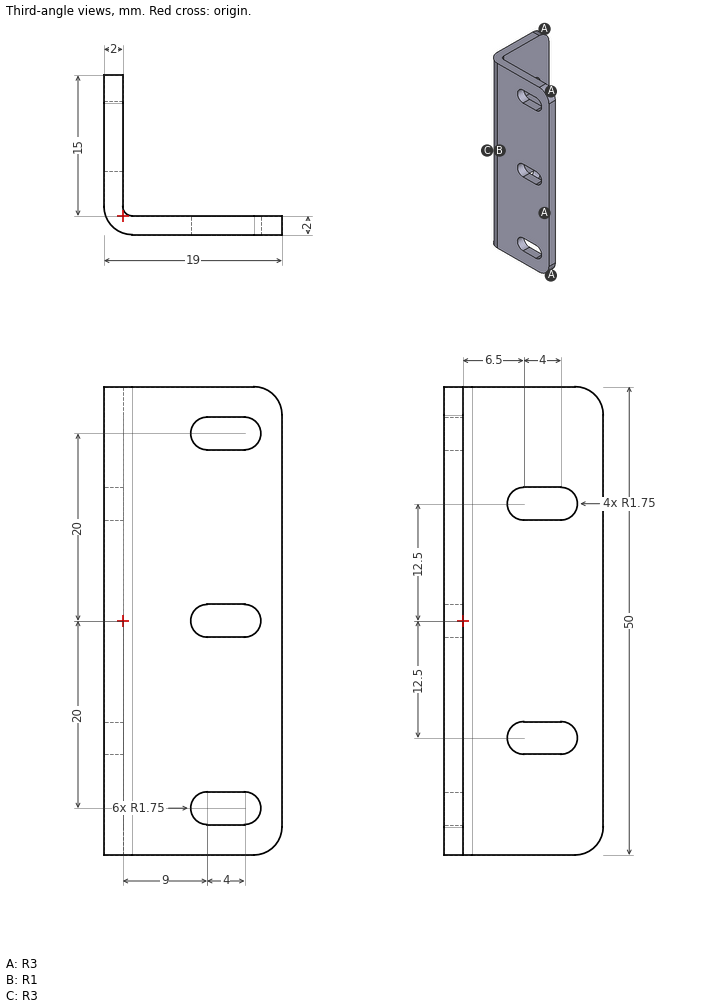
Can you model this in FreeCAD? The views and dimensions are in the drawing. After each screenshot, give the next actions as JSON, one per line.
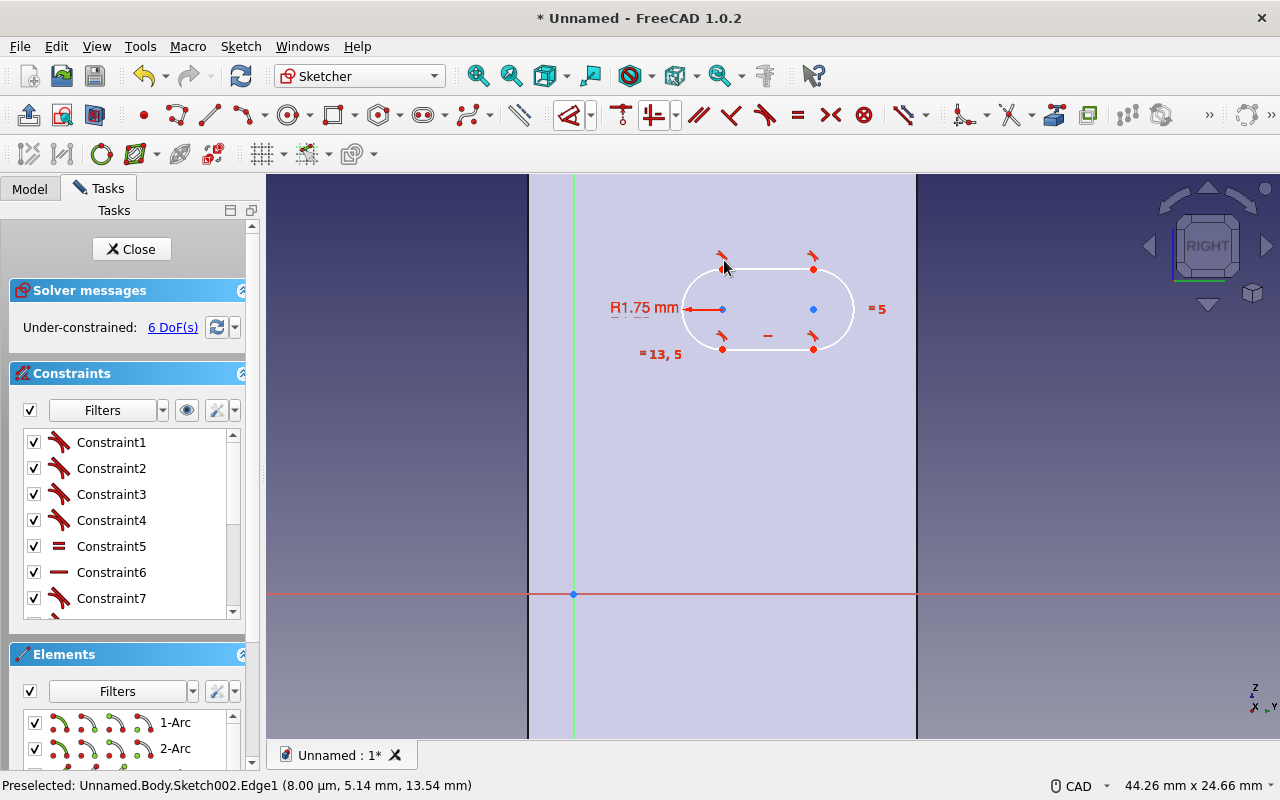
{"action": "left_click", "coordinate": [750, 269]}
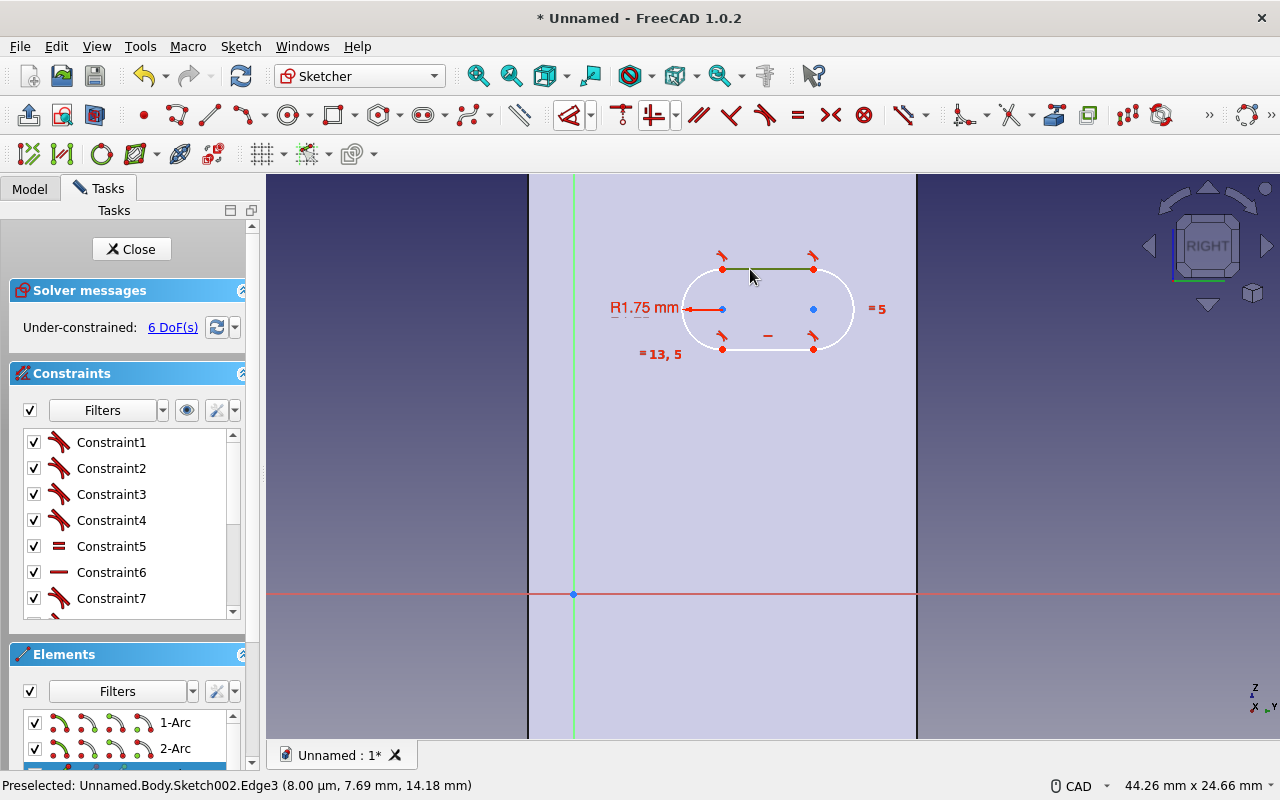
{"action": "left_click", "coordinate": [590, 116]}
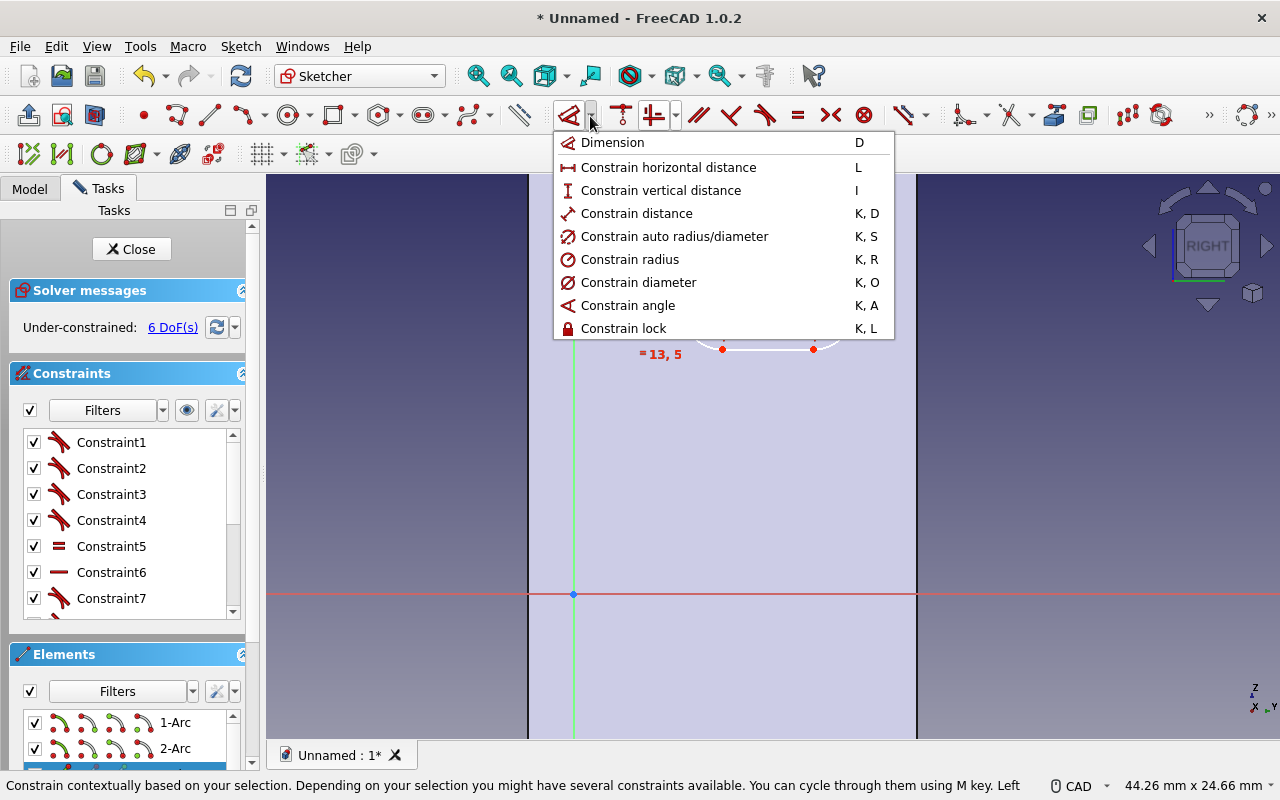
{"action": "left_click", "coordinate": [724, 168]}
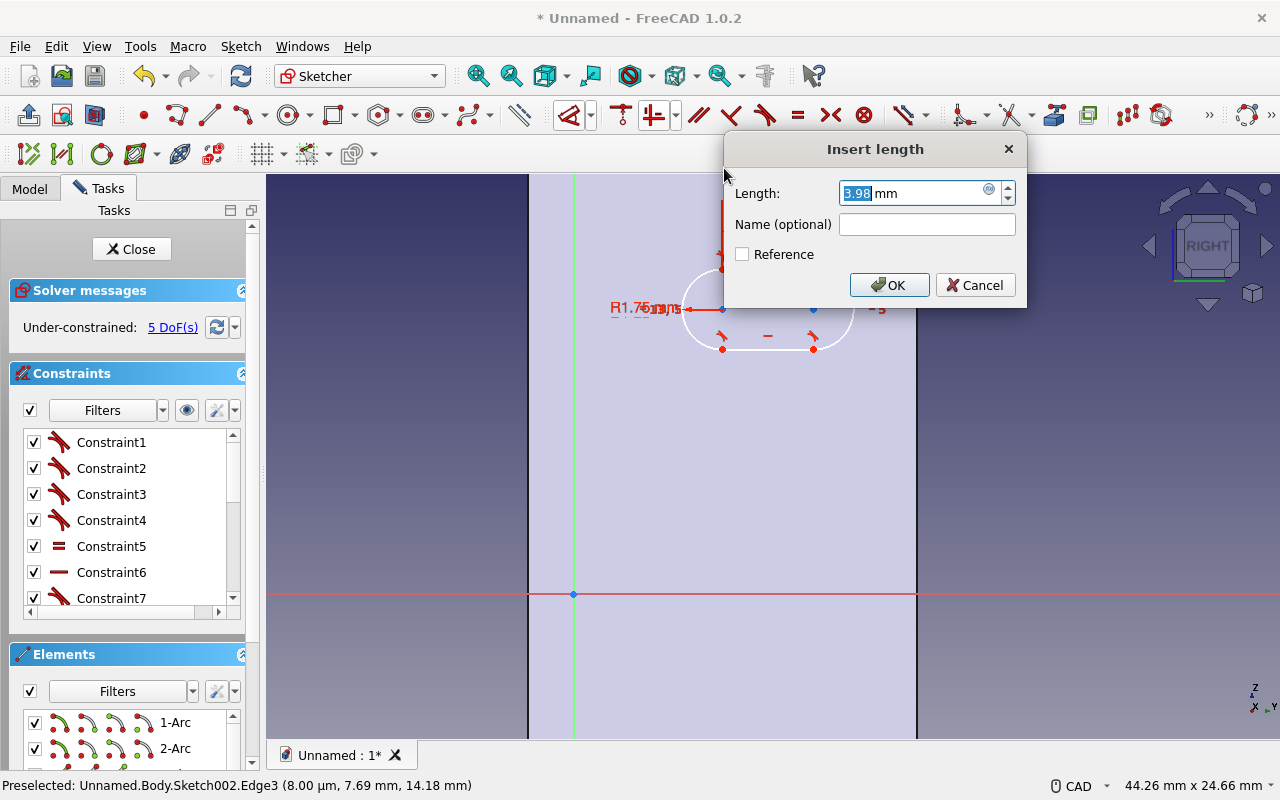
{"action": "type", "text": "4"}
{"action": "key", "text": "Return"}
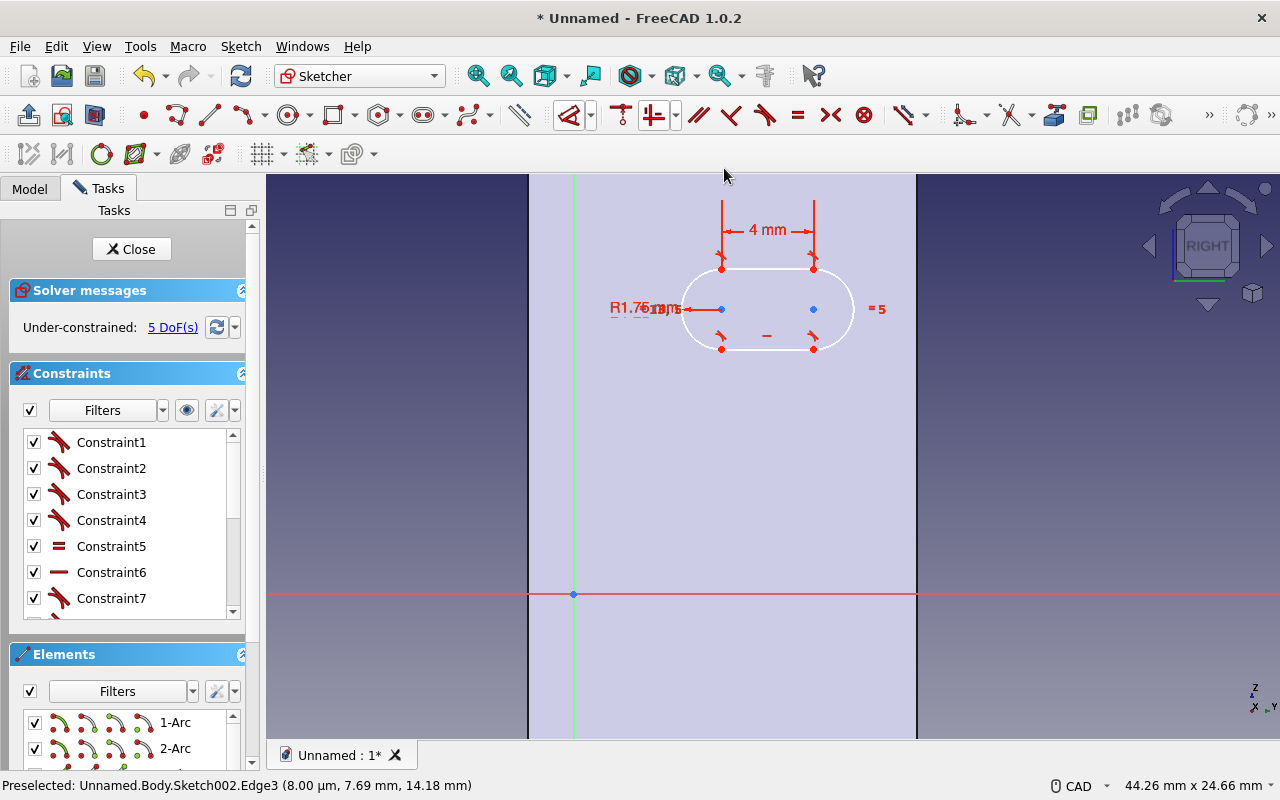
{"action": "scroll", "coordinate": [693, 289], "scroll_direction": "down", "scroll_amount": 3}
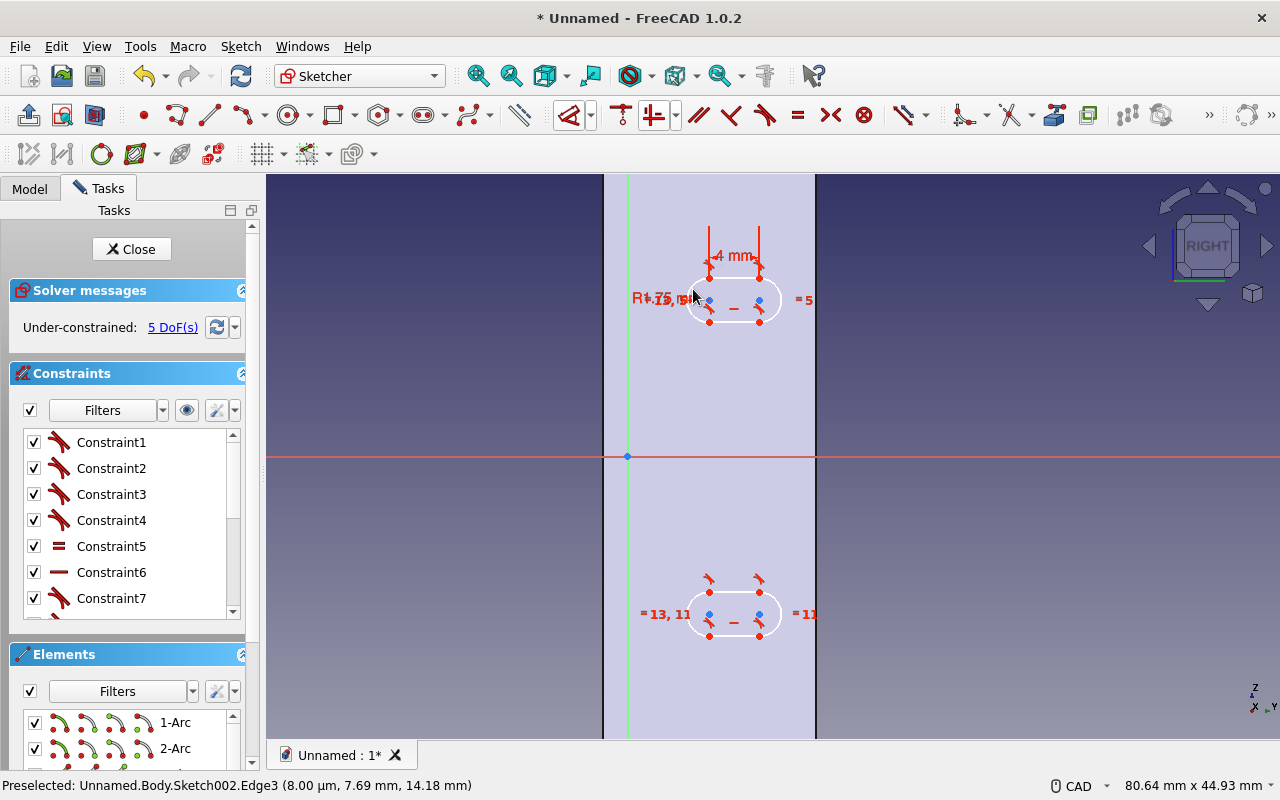
{"action": "left_click", "coordinate": [724, 592]}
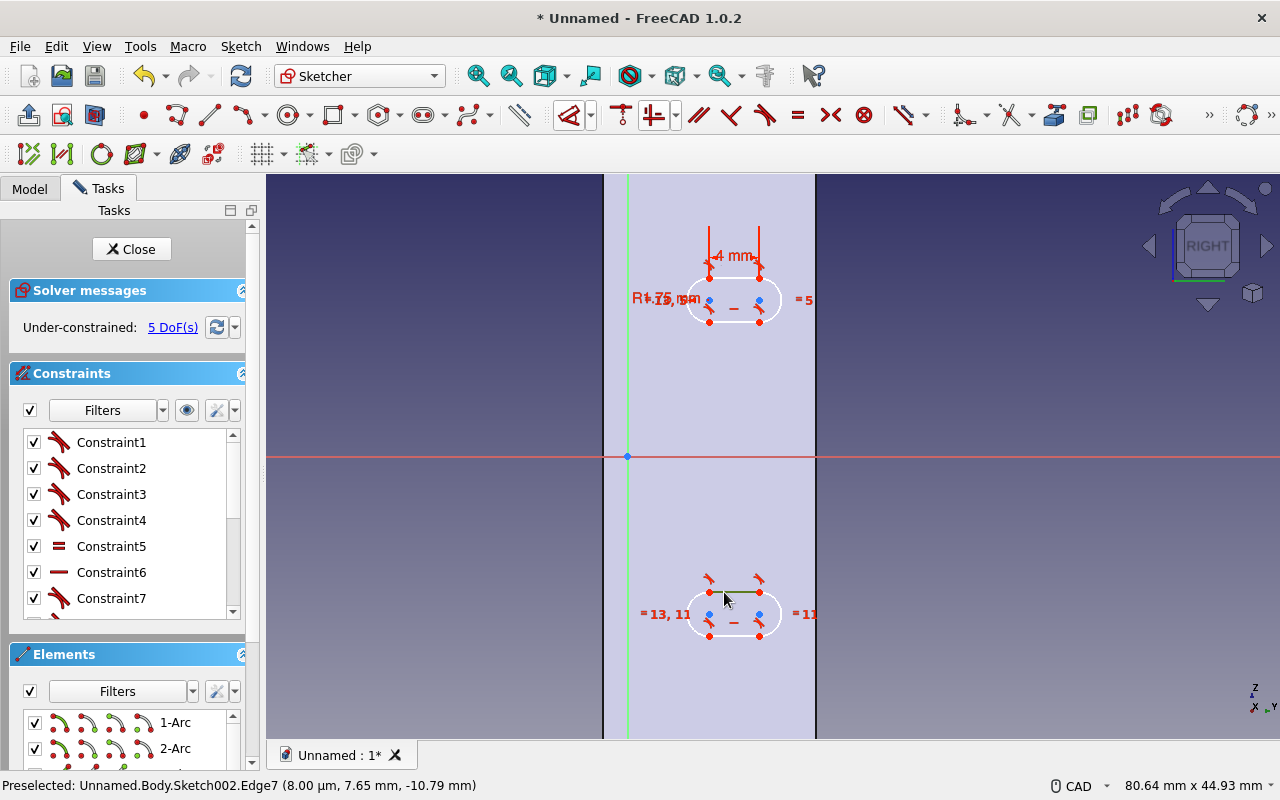
{"action": "key", "text": "l"}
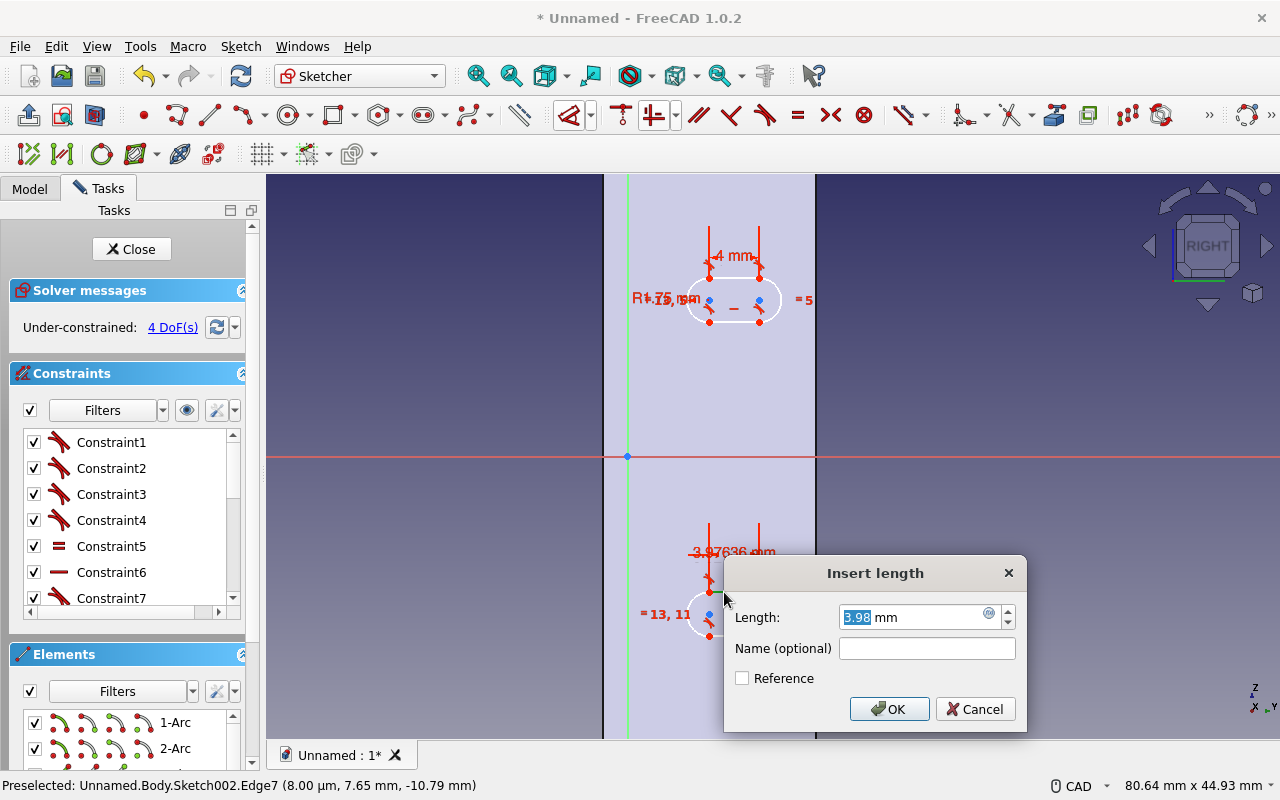
{"action": "type", "text": "4"}
{"action": "key", "text": "Return"}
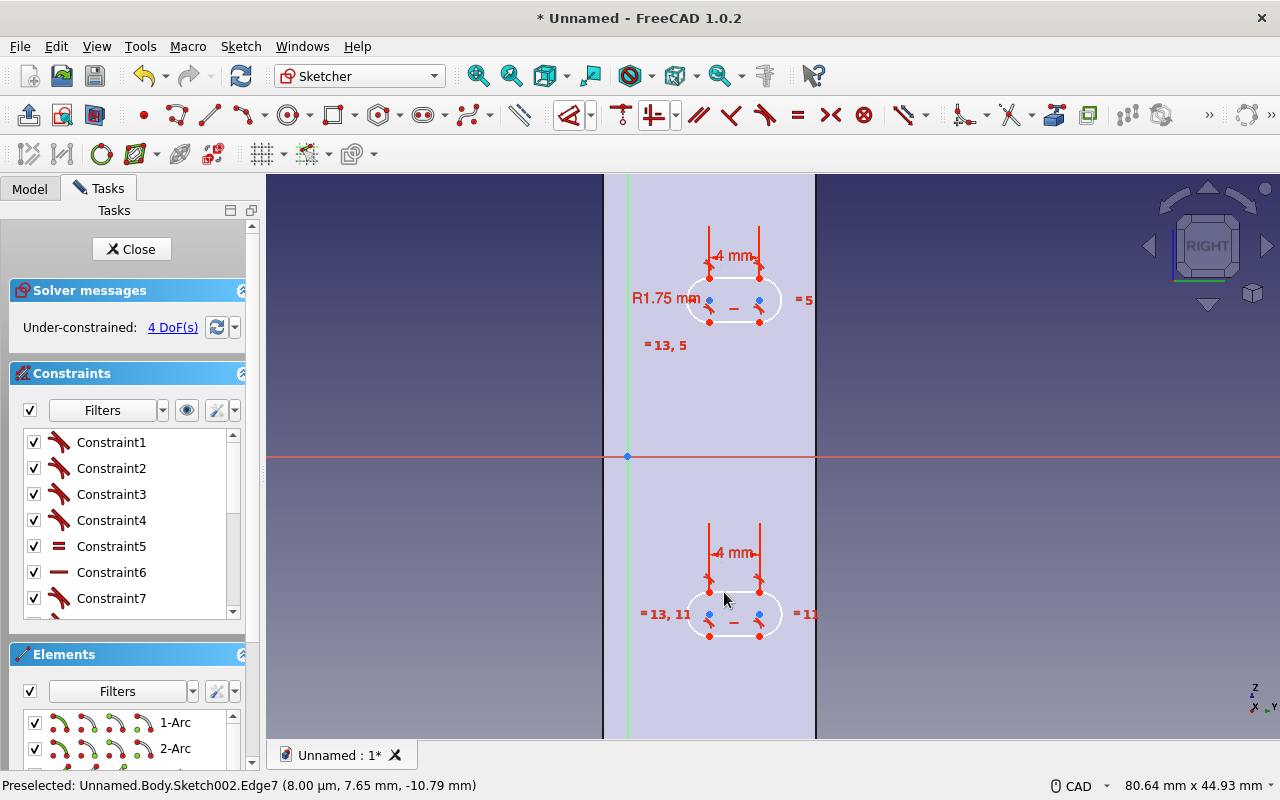
{"action": "left_click", "coordinate": [709, 278]}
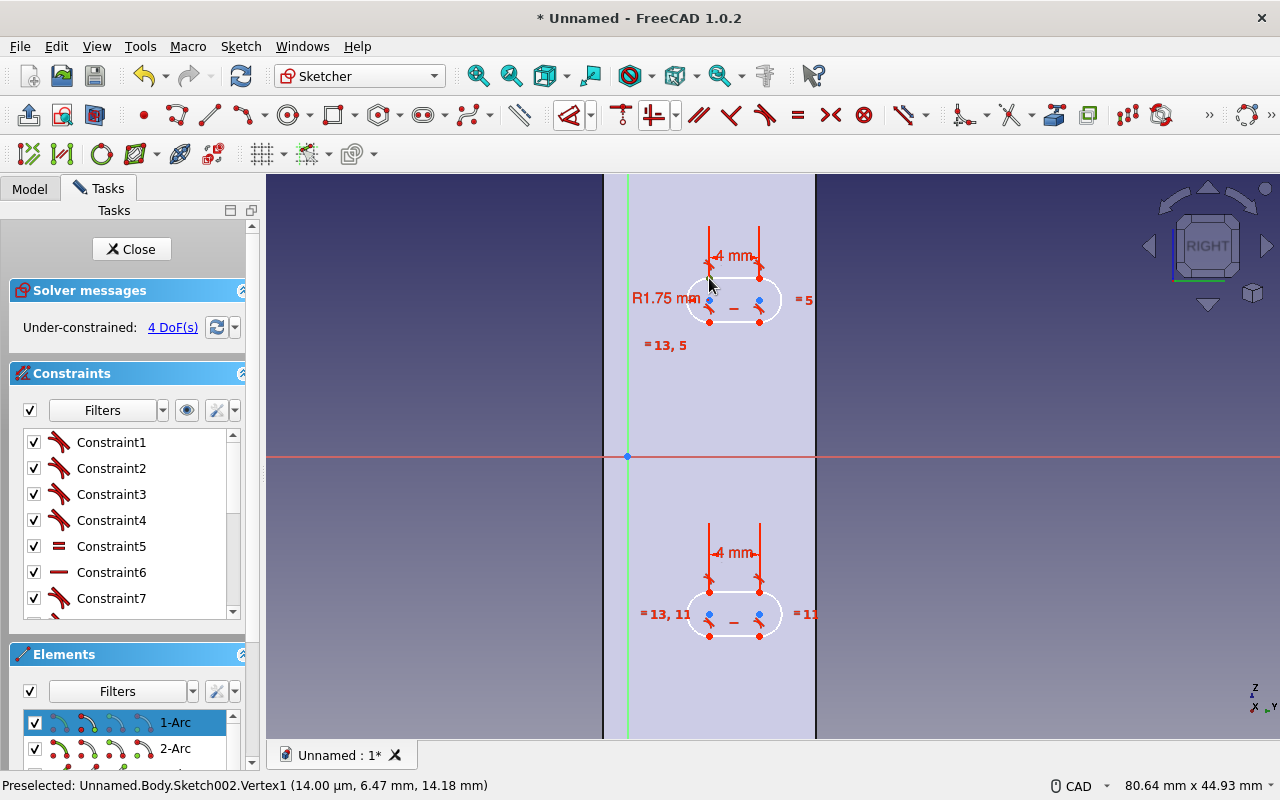
{"action": "key", "text": "l"}